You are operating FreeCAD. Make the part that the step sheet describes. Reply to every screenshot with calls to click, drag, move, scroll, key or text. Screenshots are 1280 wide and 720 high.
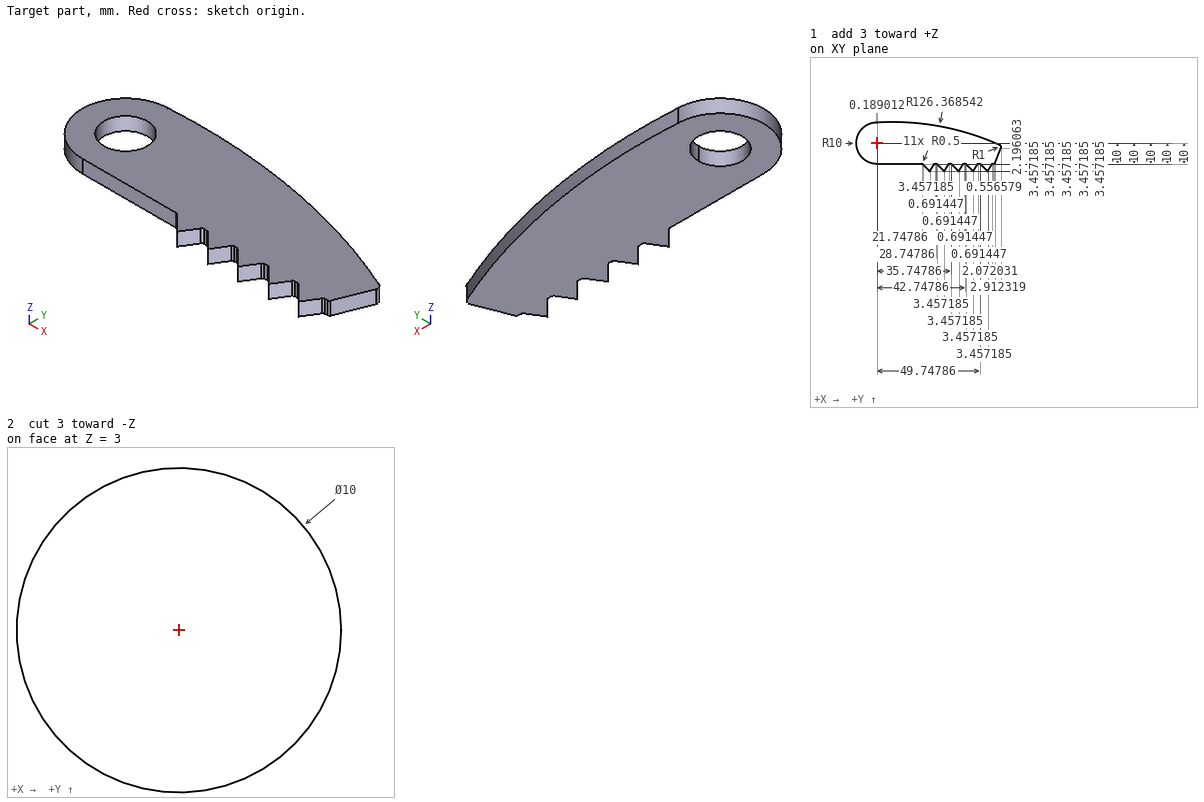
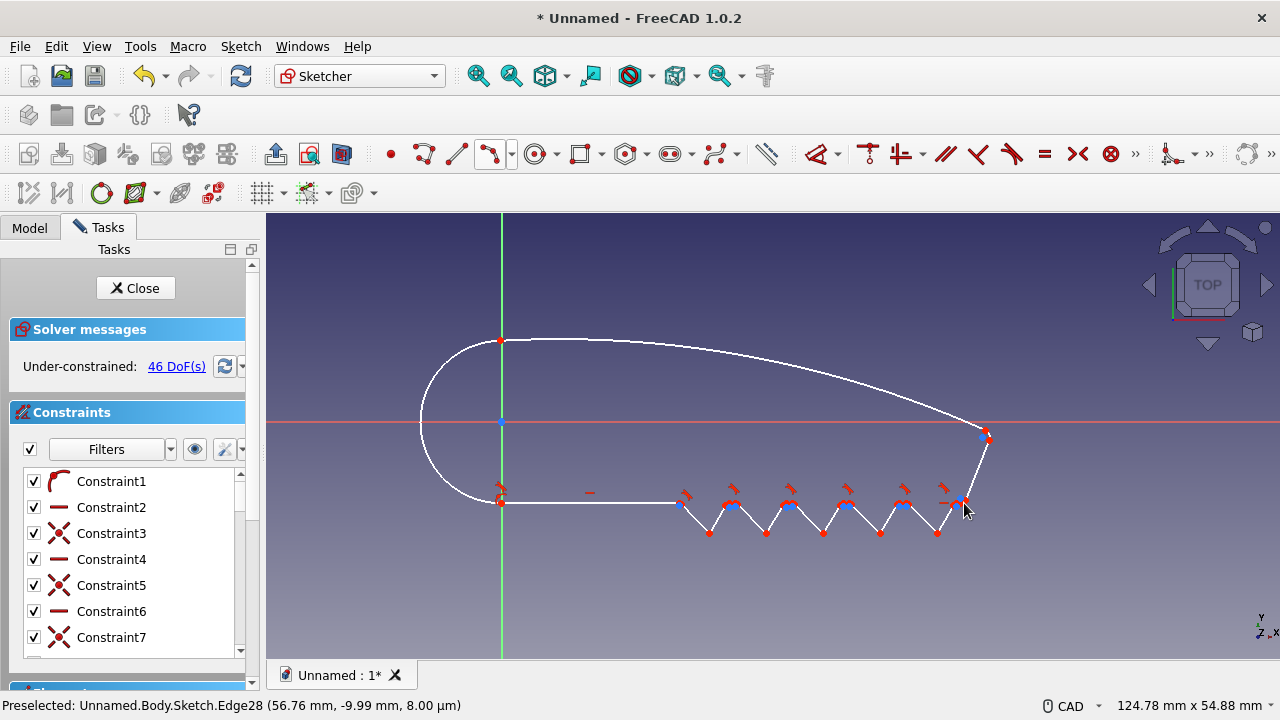
click(973, 482)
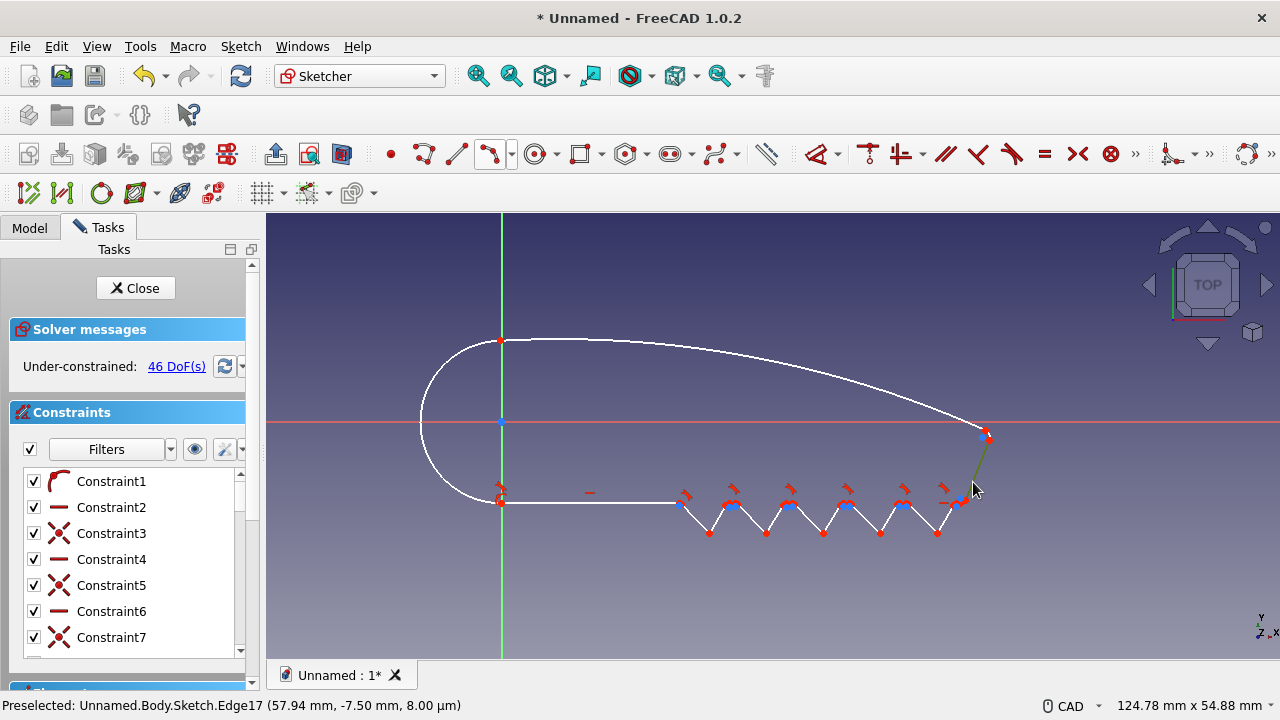
scroll(989, 434, up, 5)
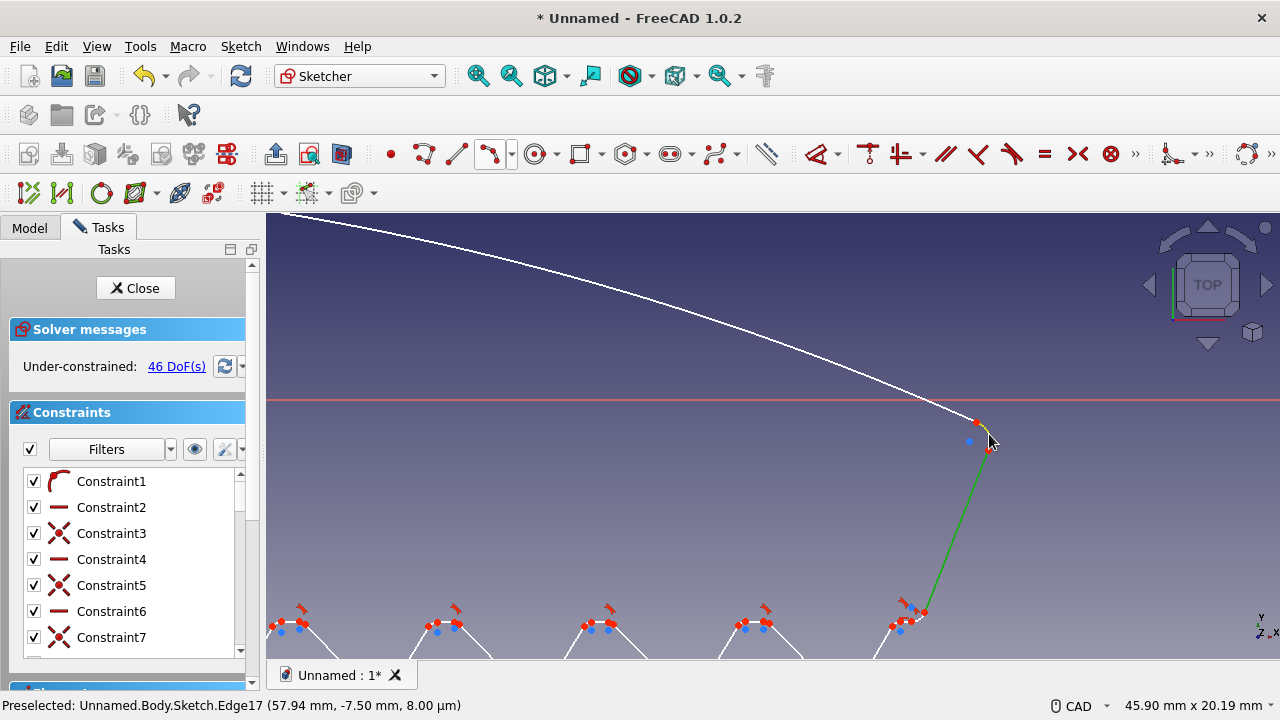
click(989, 434)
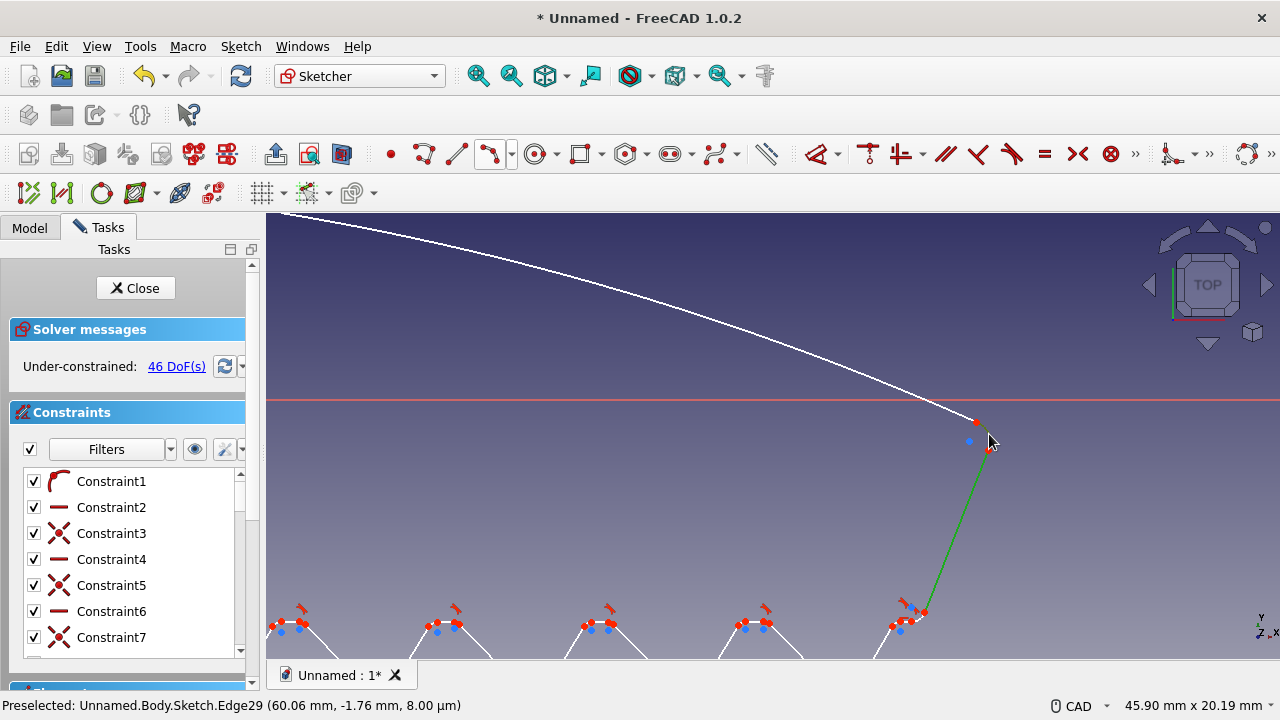
click(1012, 154)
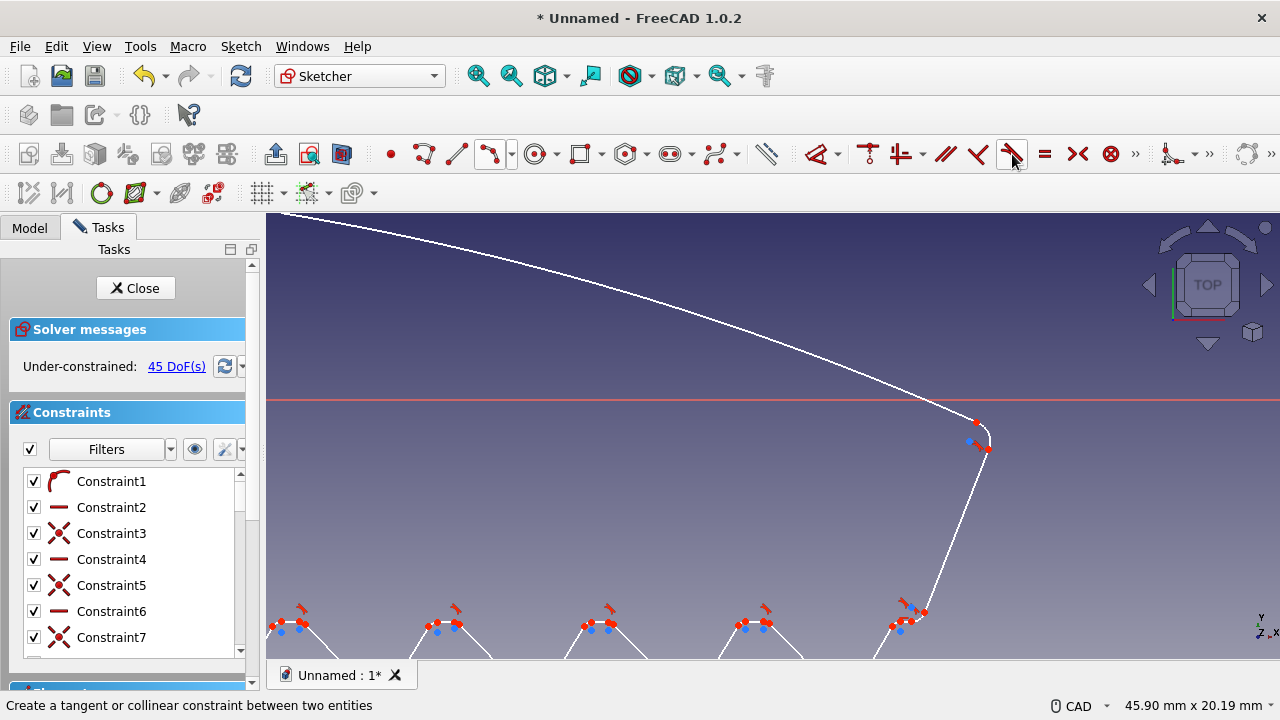
scroll(990, 440, up, 2)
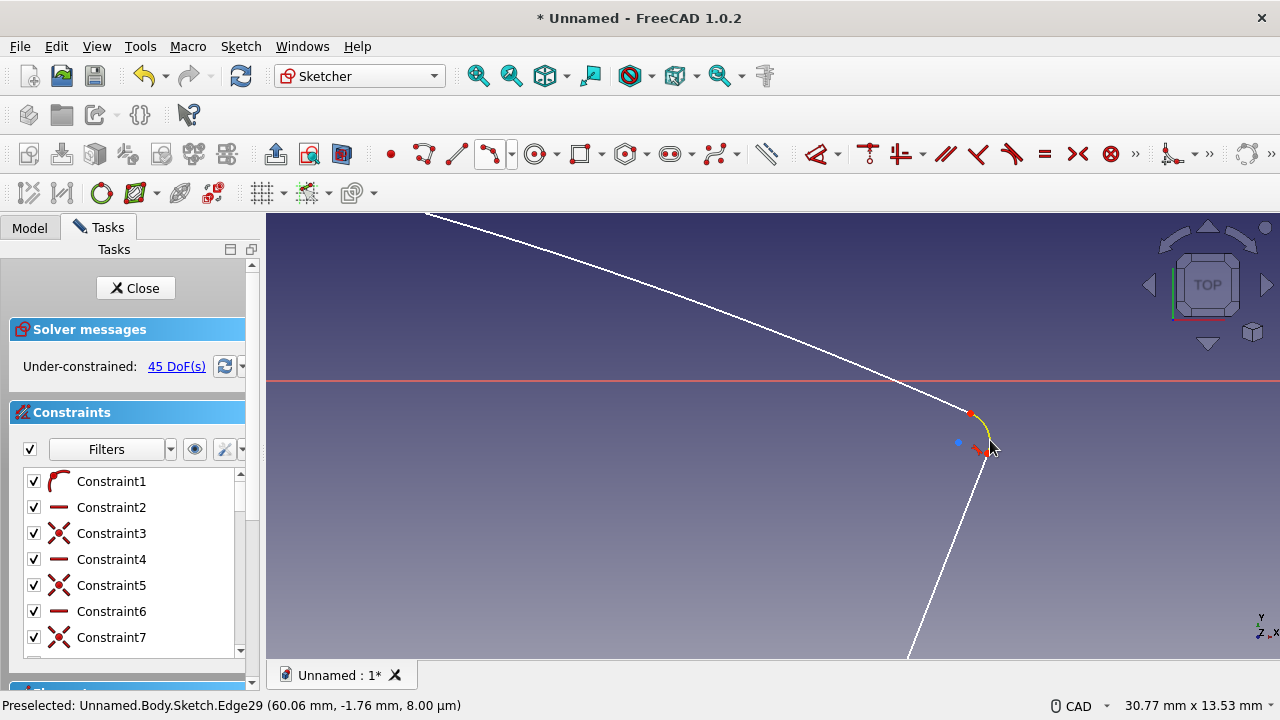
click(990, 439)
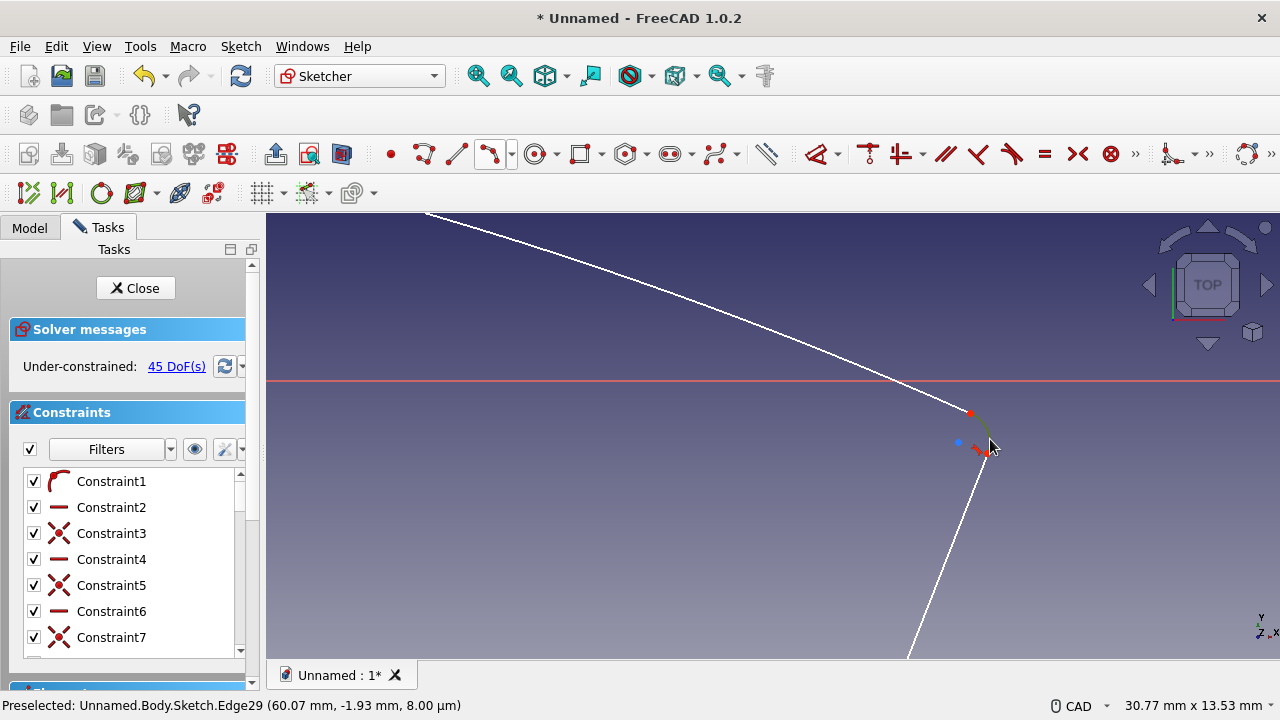
scroll(989, 435, down, 7)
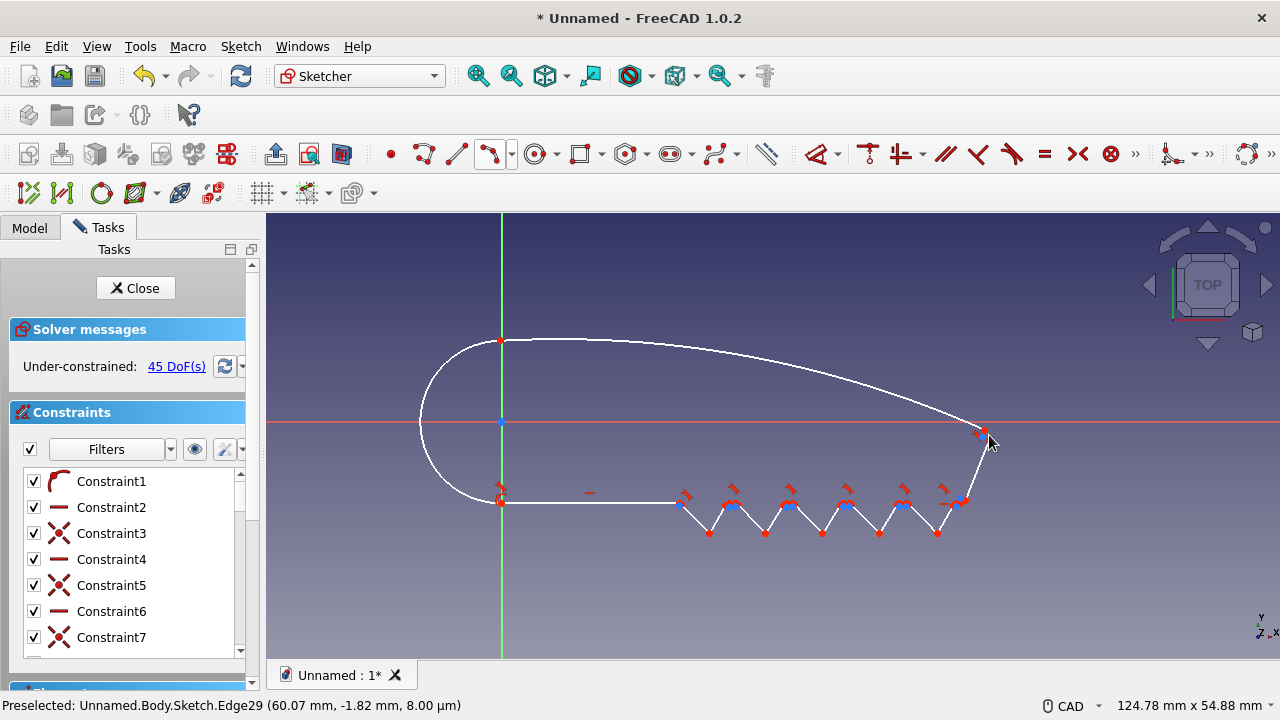
click(892, 394)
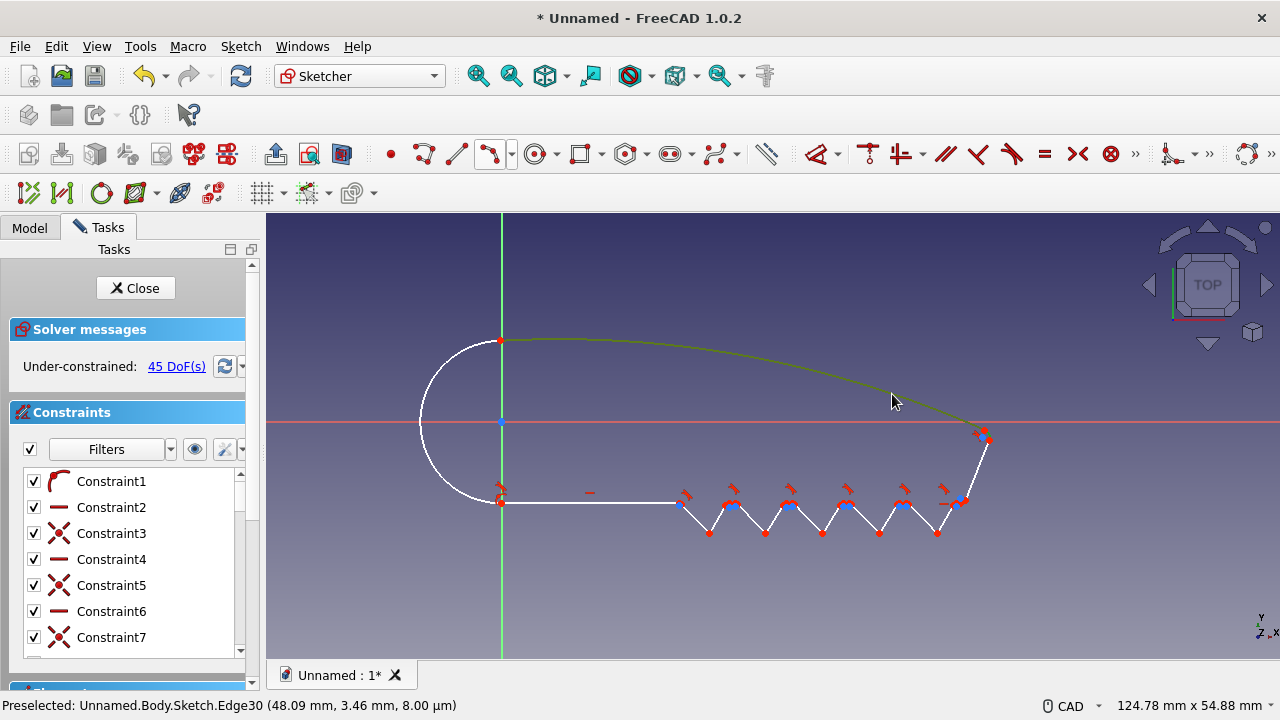
key(t)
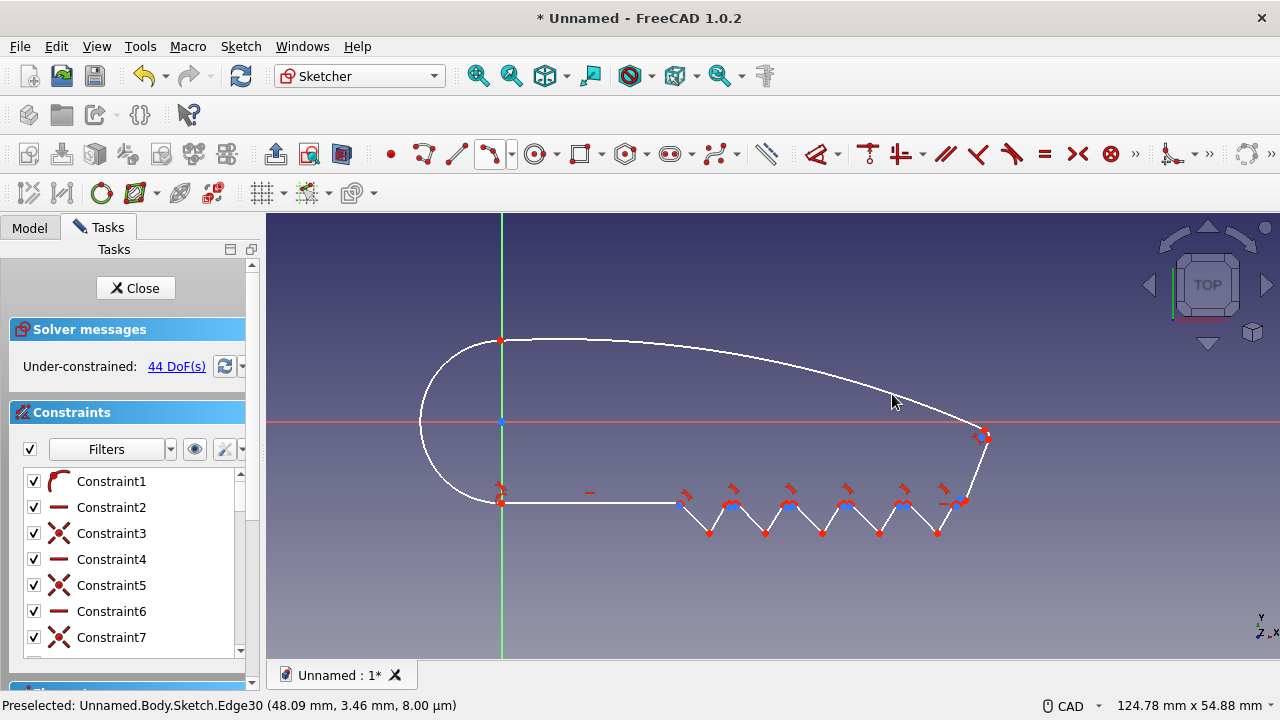
scroll(680, 504, up, 13)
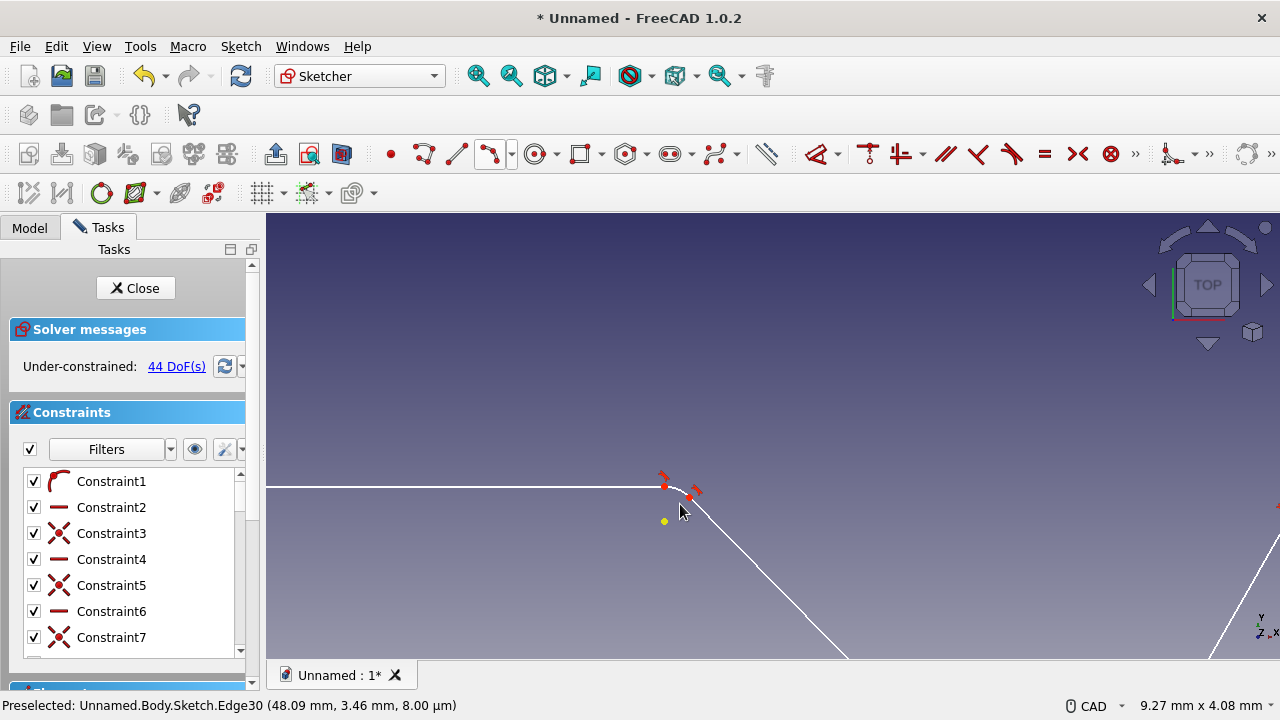
click(678, 489)